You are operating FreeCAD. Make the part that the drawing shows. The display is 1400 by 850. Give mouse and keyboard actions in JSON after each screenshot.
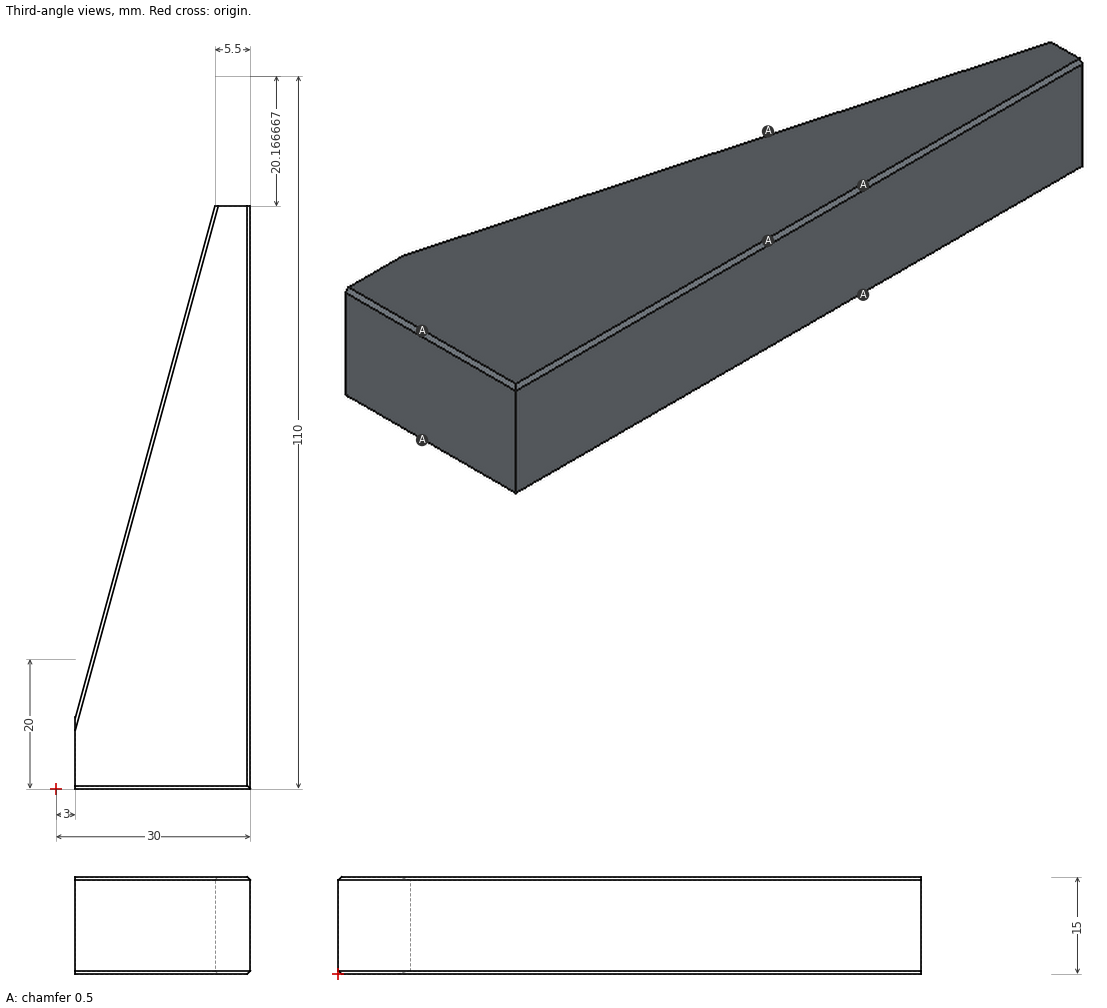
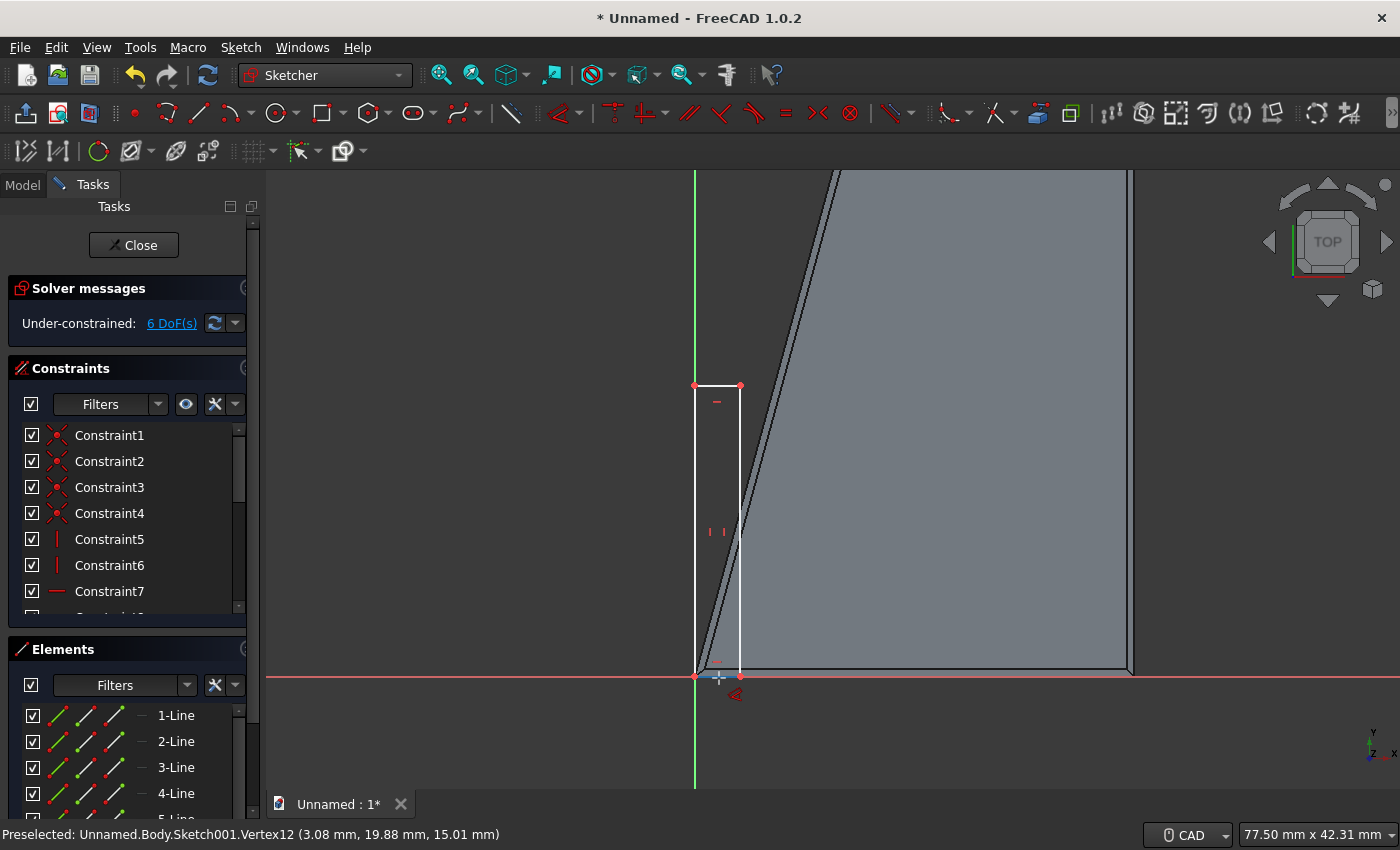
{"action": "left_click", "coordinate": [718, 677]}
{"action": "left_click", "coordinate": [718, 711]}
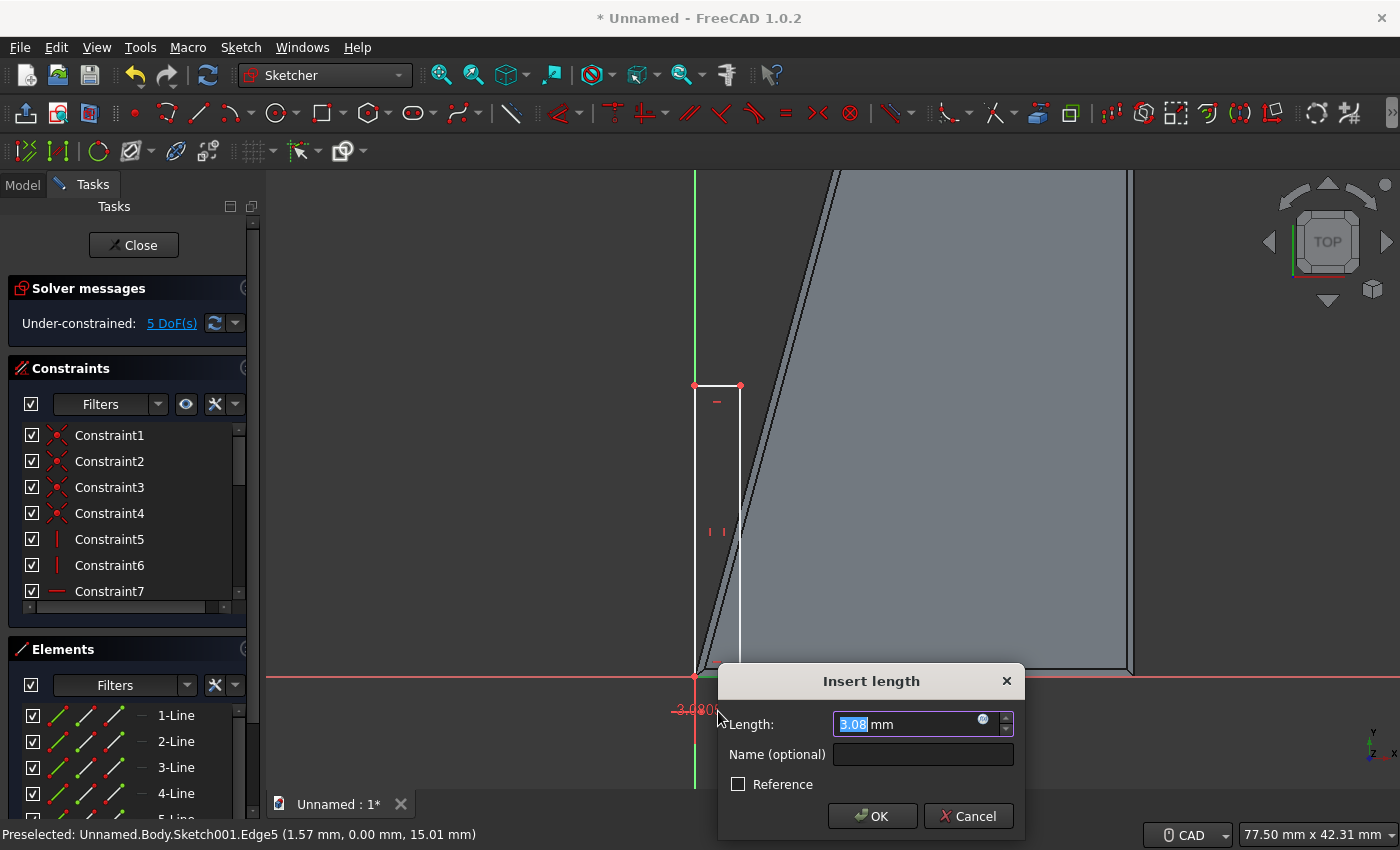
{"action": "type", "text": "3"}
{"action": "key", "text": "Return"}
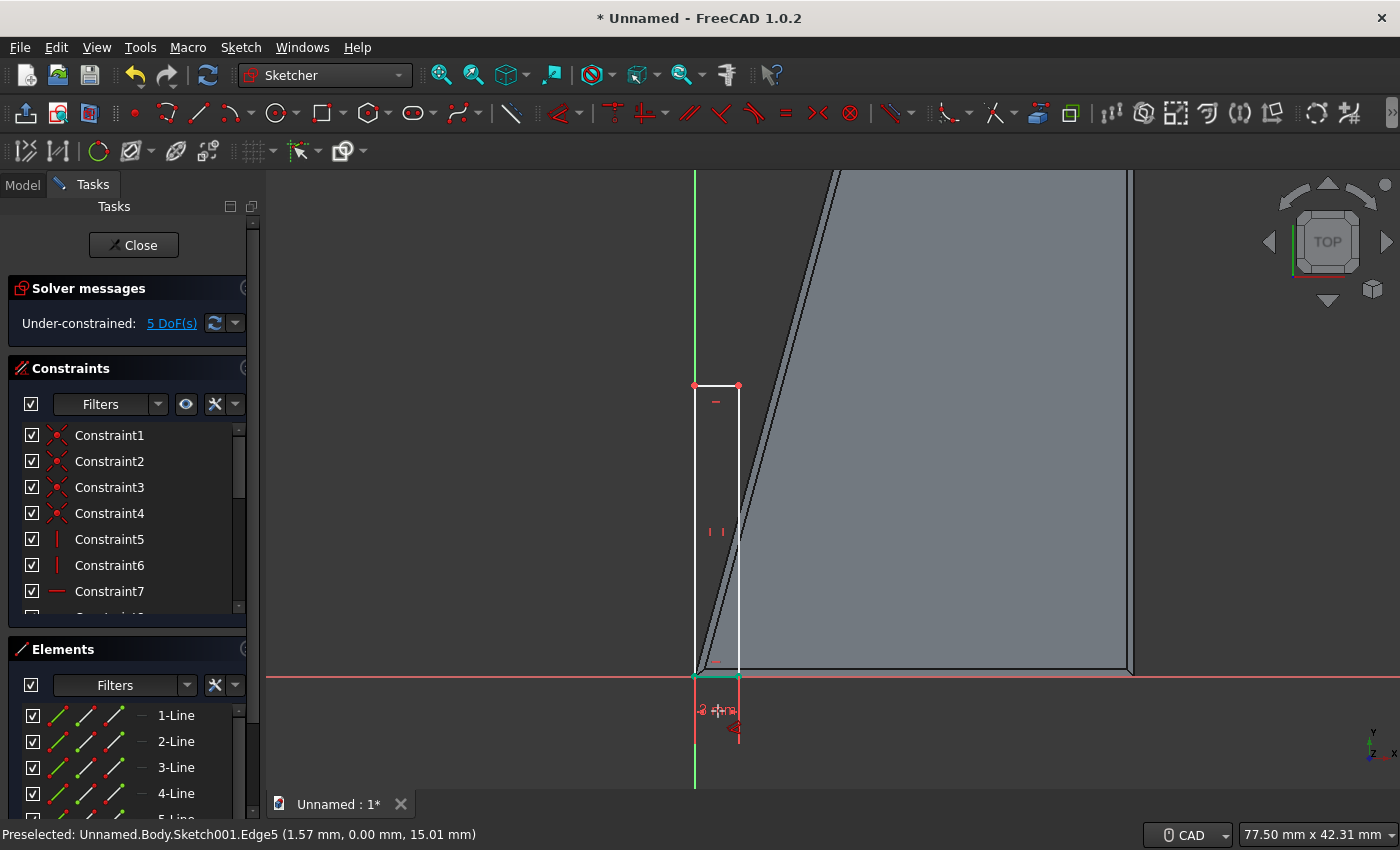
{"action": "scroll", "coordinate": [715, 678], "scroll_direction": "down", "scroll_amount": 7}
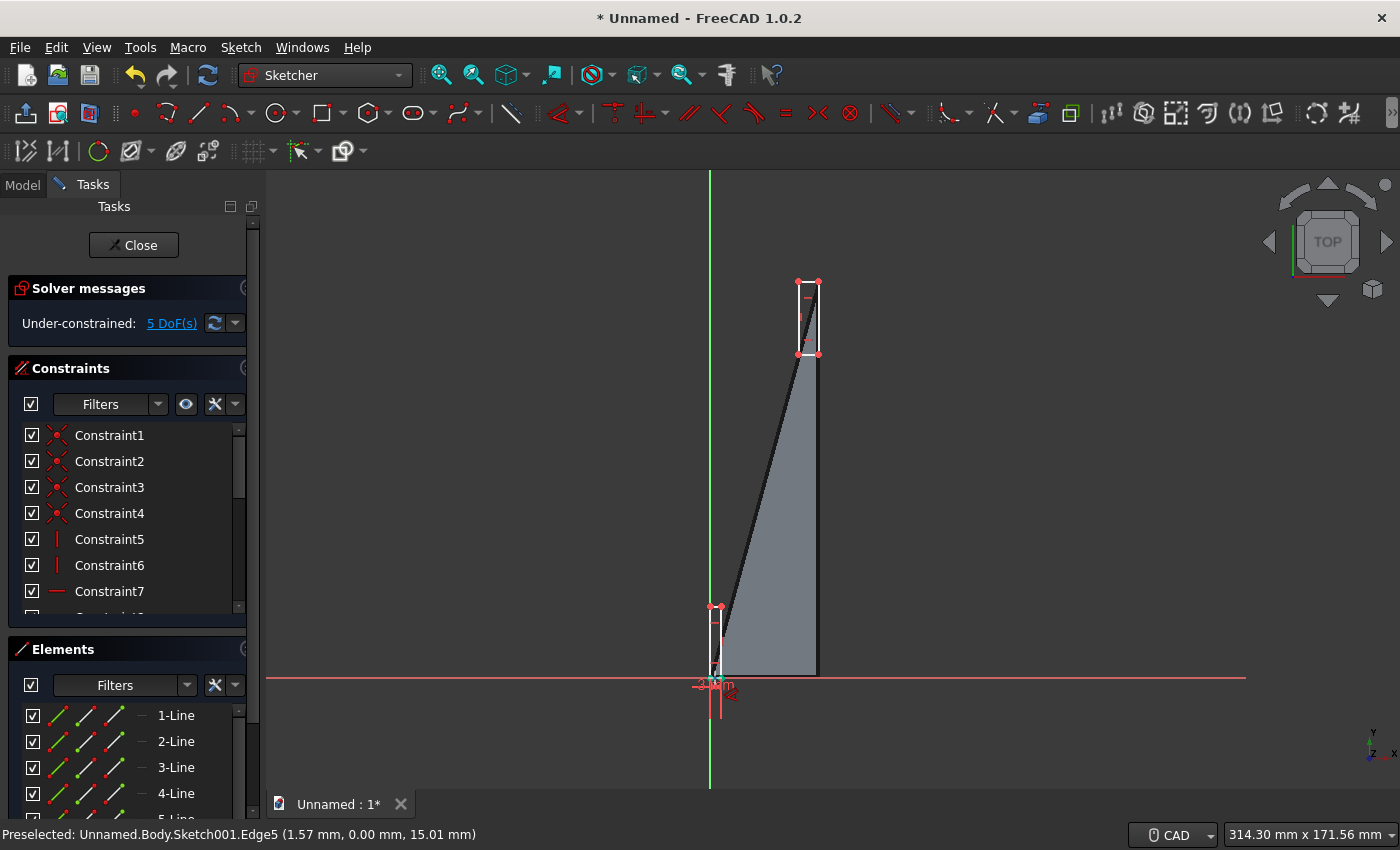
{"action": "scroll", "coordinate": [721, 657], "scroll_direction": "up", "scroll_amount": 2}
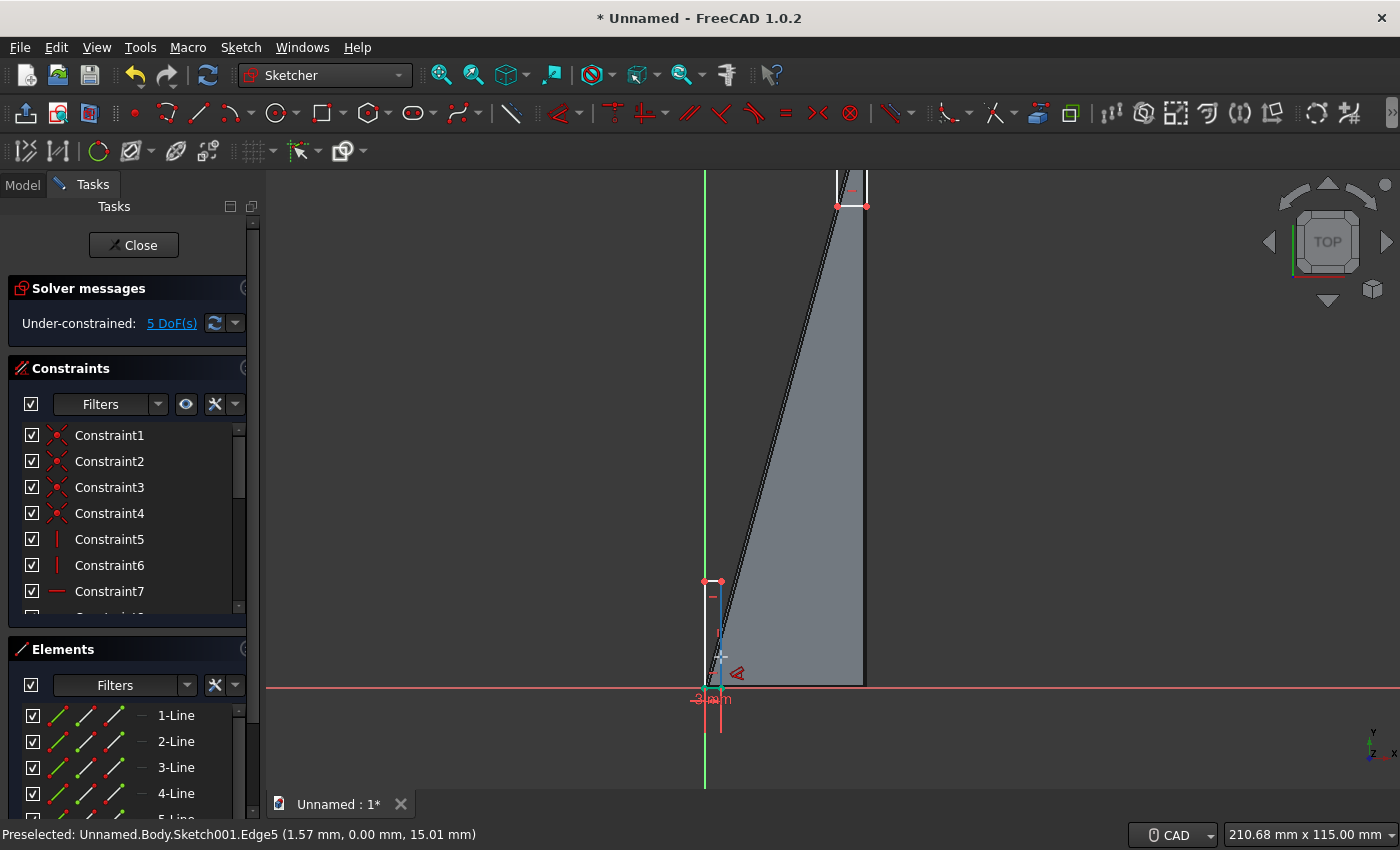
{"action": "left_click", "coordinate": [721, 656]}
{"action": "left_click", "coordinate": [687, 635]}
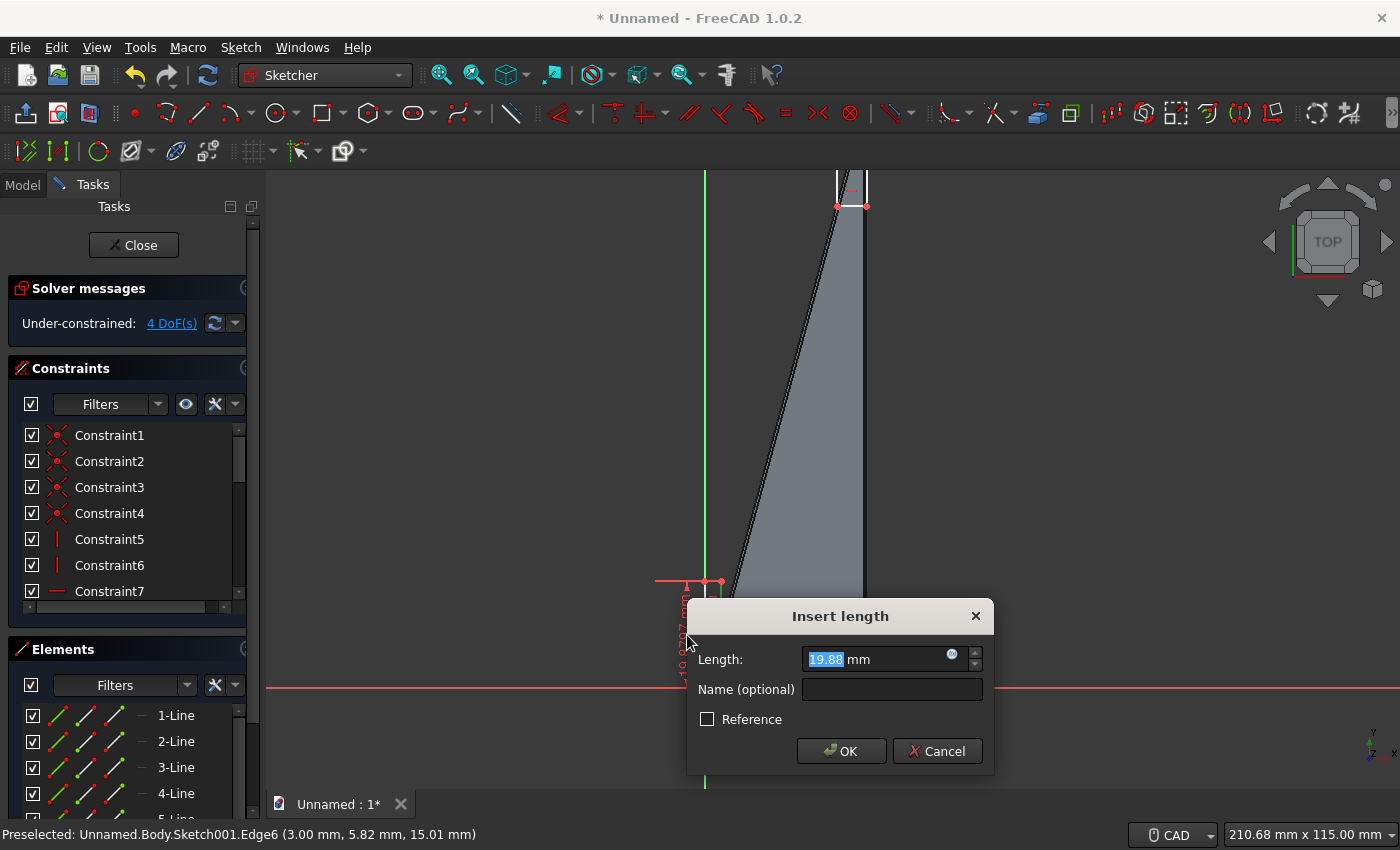
{"action": "type", "text": "20"}
{"action": "key", "text": "Return"}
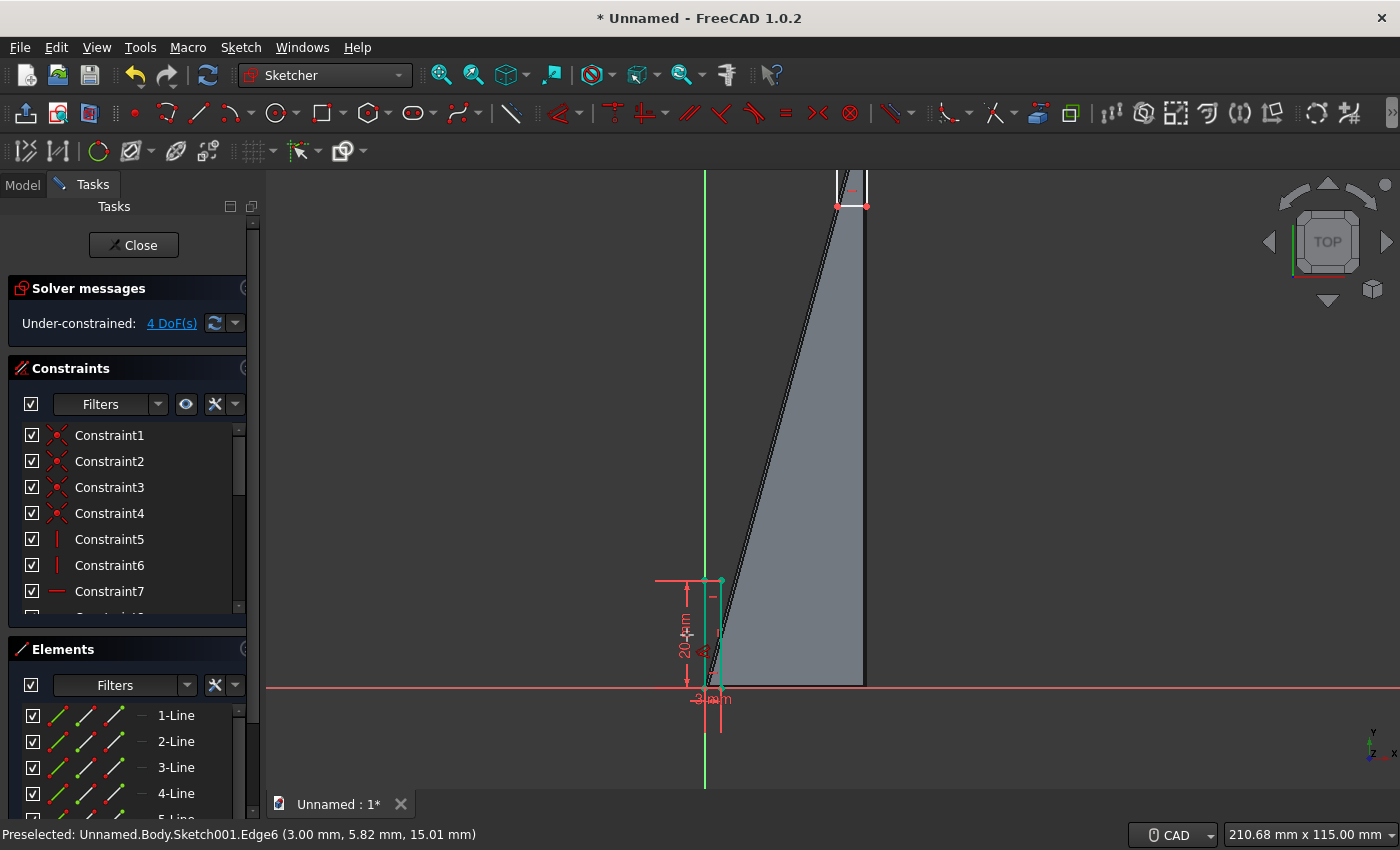
{"action": "scroll", "coordinate": [849, 206], "scroll_direction": "up", "scroll_amount": 2}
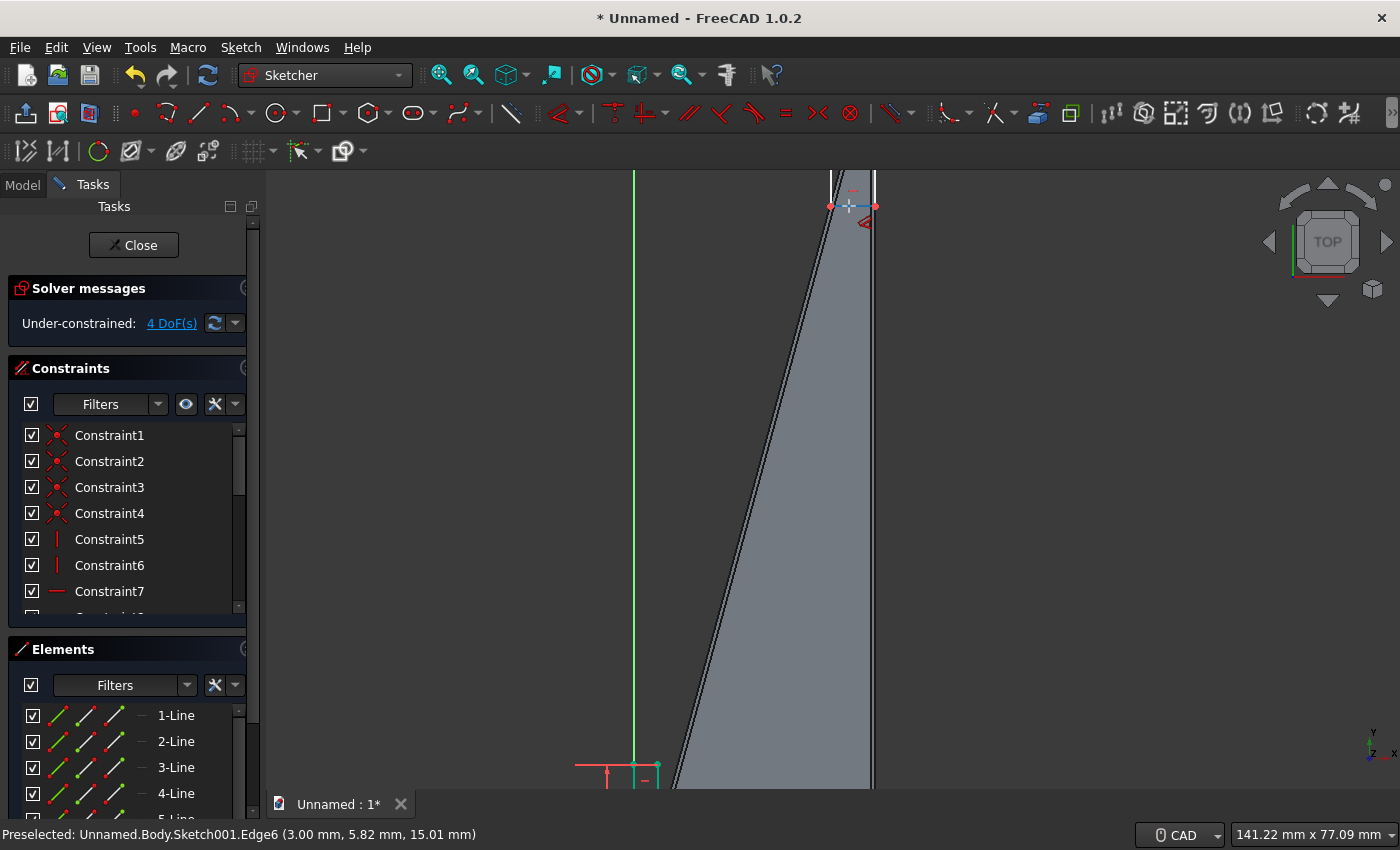
{"action": "left_click", "coordinate": [849, 206]}
{"action": "left_click", "coordinate": [853, 240]}